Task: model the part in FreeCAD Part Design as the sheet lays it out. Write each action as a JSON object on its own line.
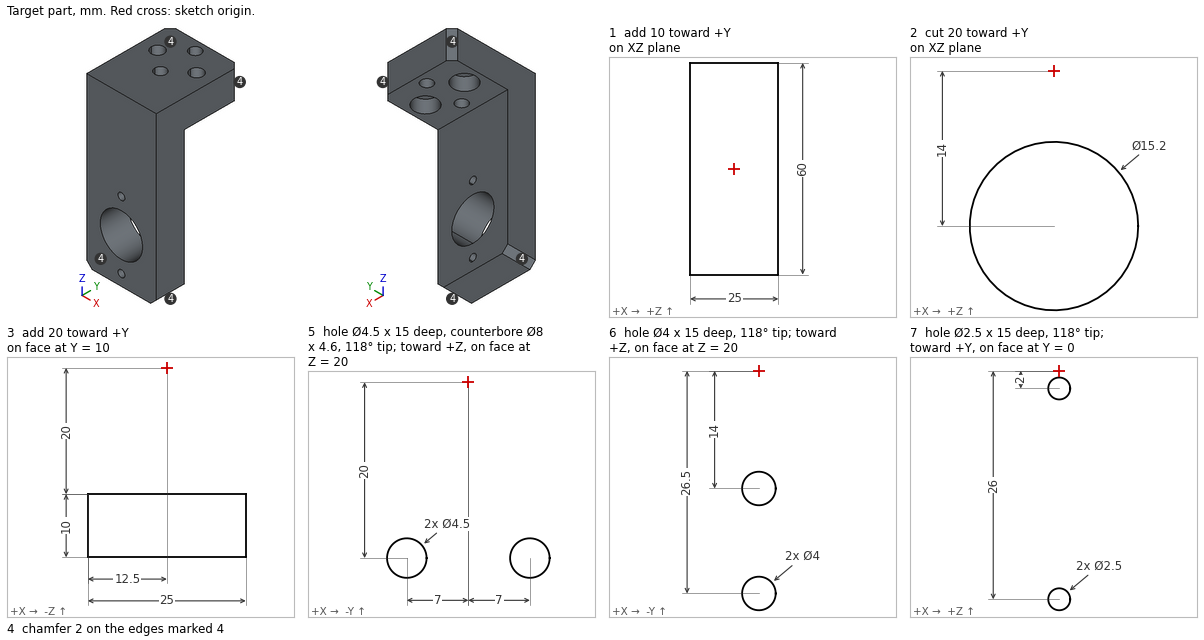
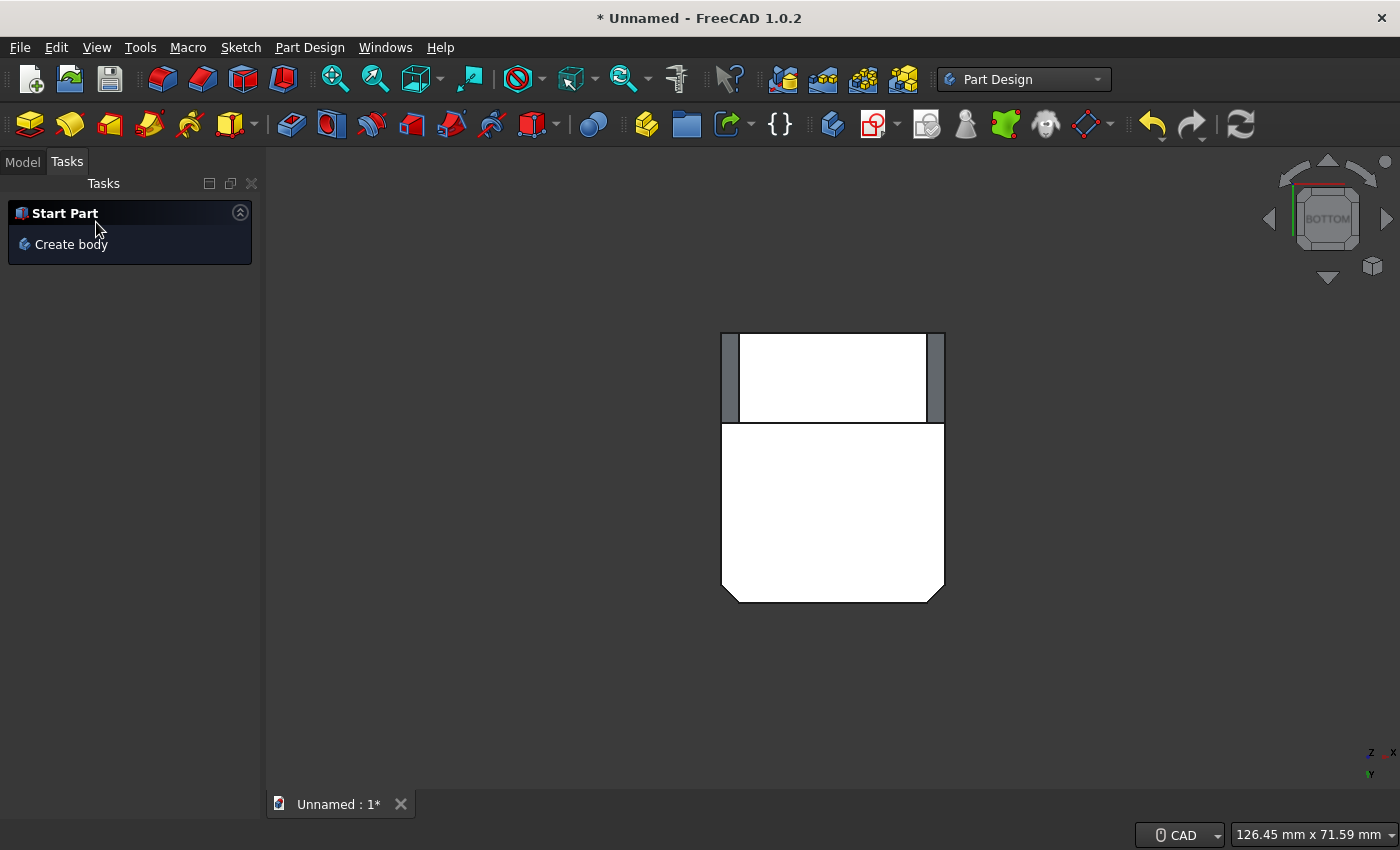
{"action": "left_click", "coordinate": [833, 512]}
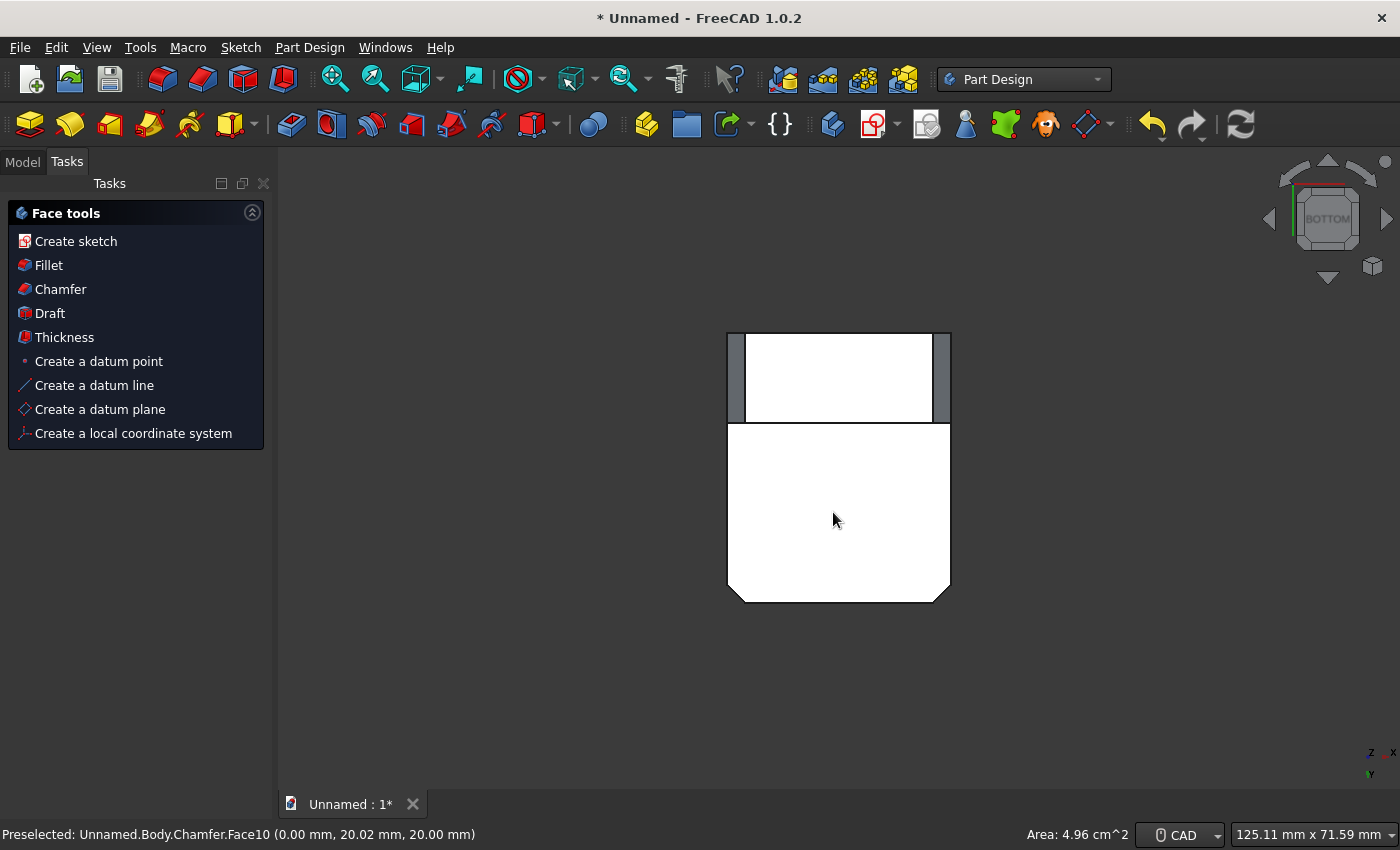
{"action": "left_click", "coordinate": [874, 124]}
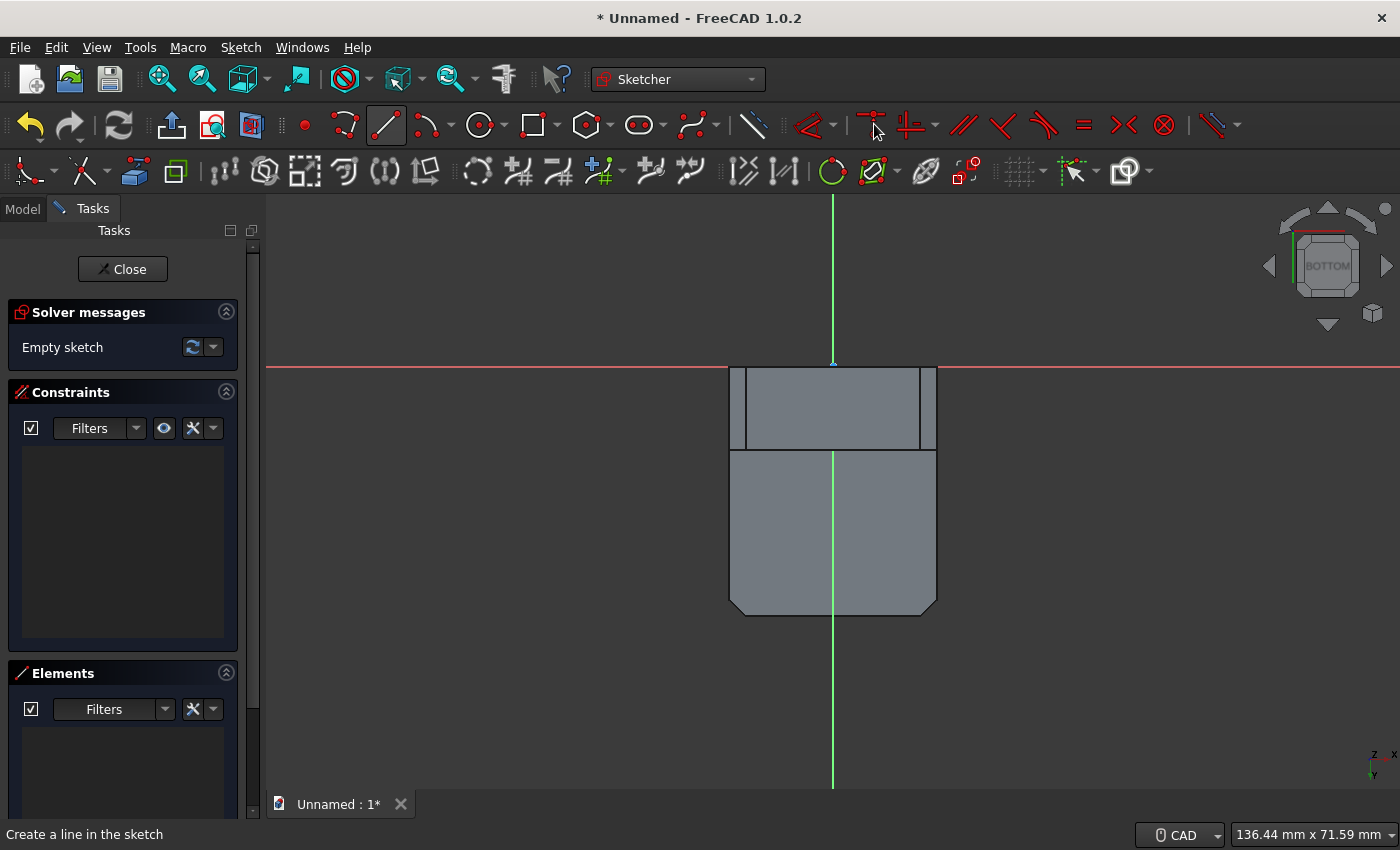
{"action": "key", "text": "q s"}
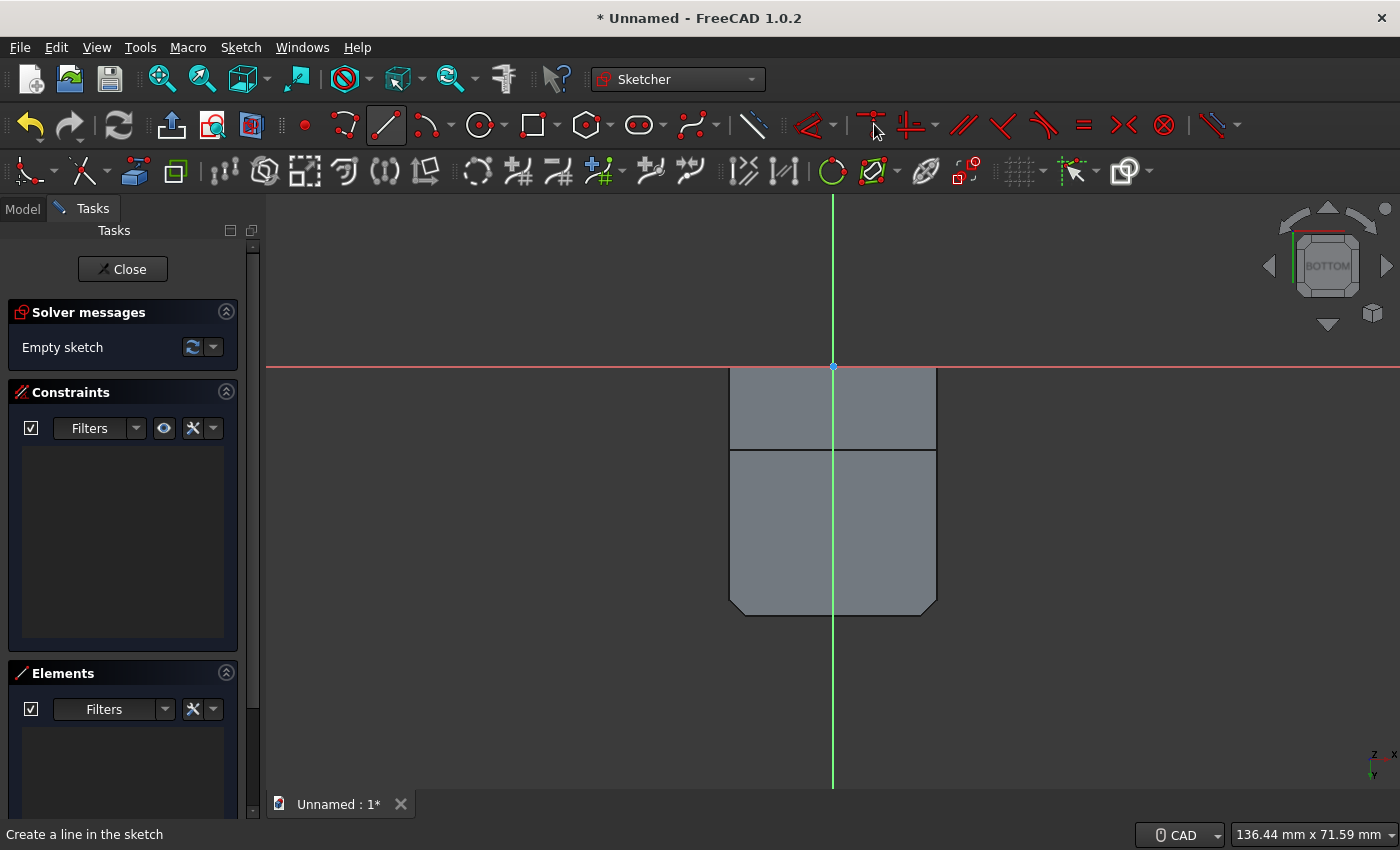
{"action": "scroll", "coordinate": [889, 433], "scroll_direction": "up", "scroll_amount": 4}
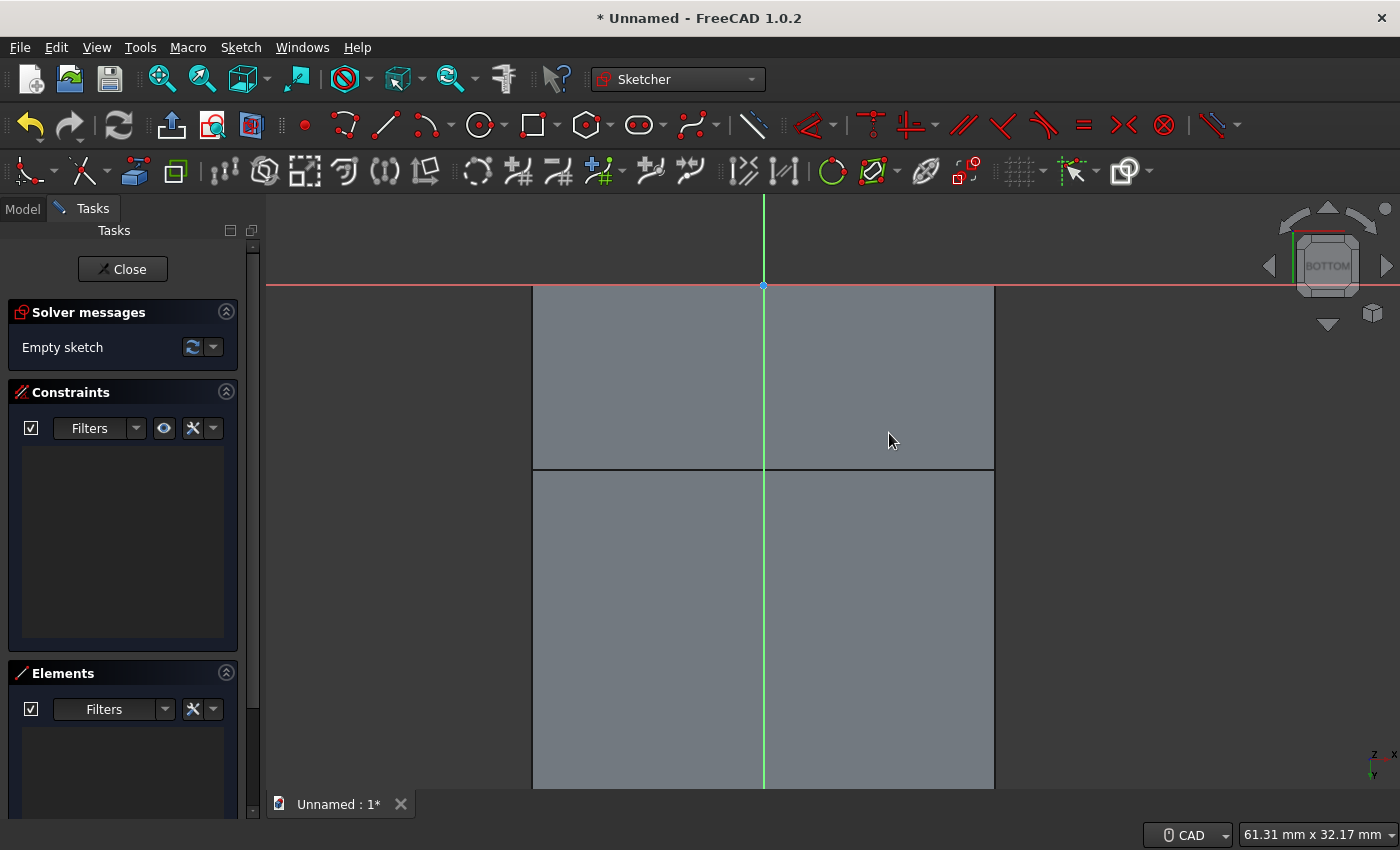
{"action": "key", "text": "g c"}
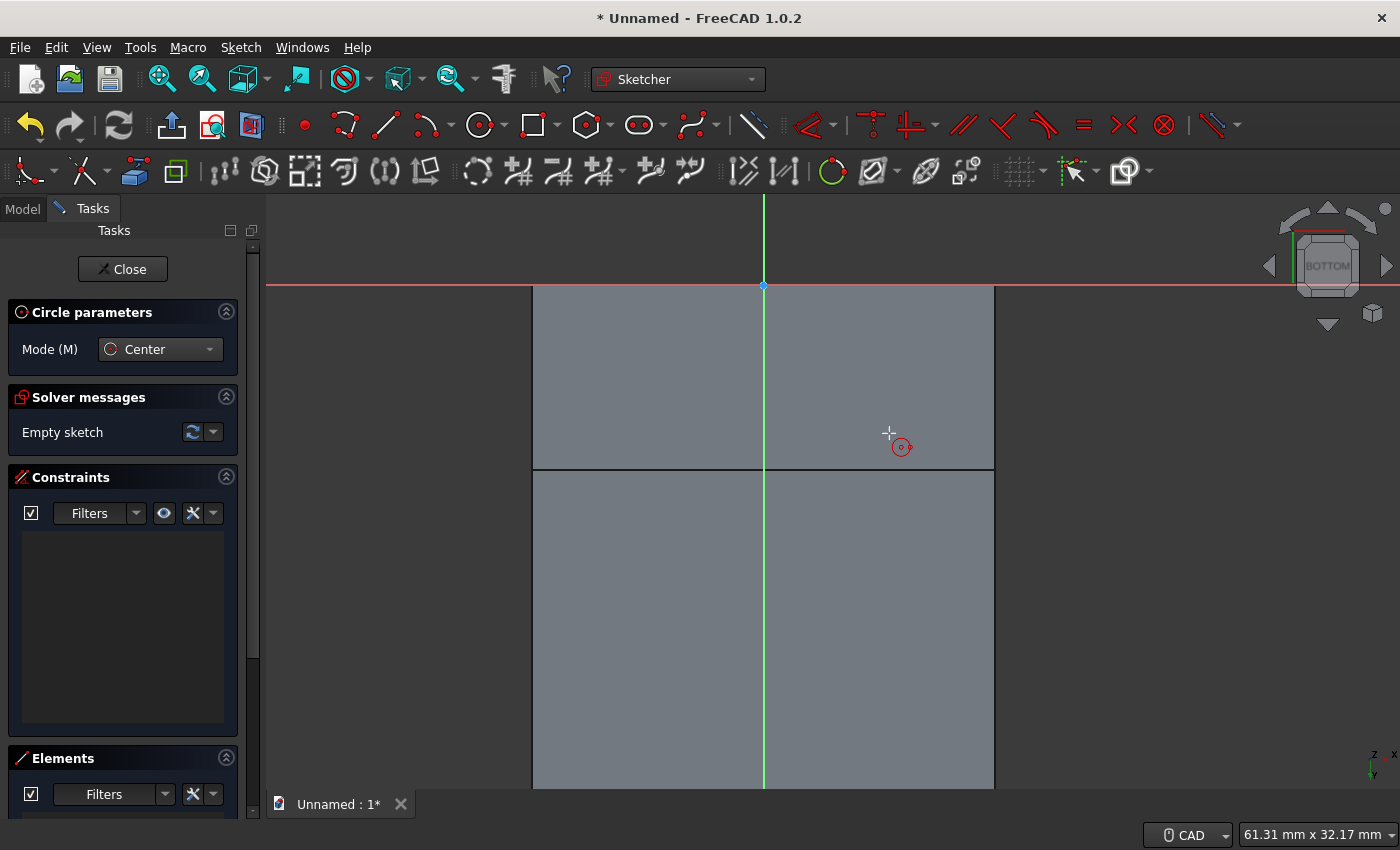
{"action": "left_click", "coordinate": [634, 655]}
{"action": "left_click", "coordinate": [664, 626]}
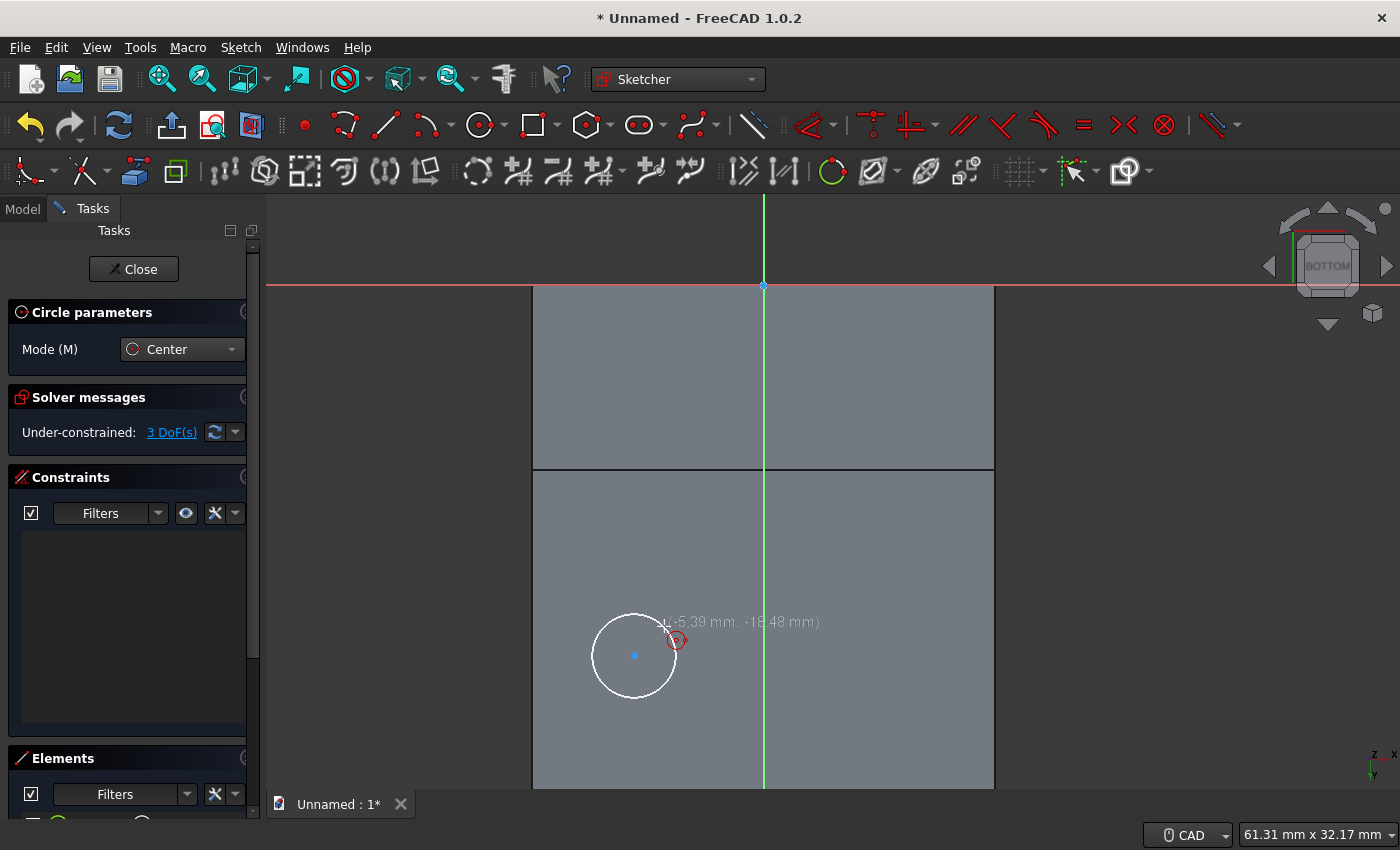
{"action": "left_click", "coordinate": [893, 655]}
{"action": "left_click", "coordinate": [923, 626]}
{"action": "key", "text": "Escape"}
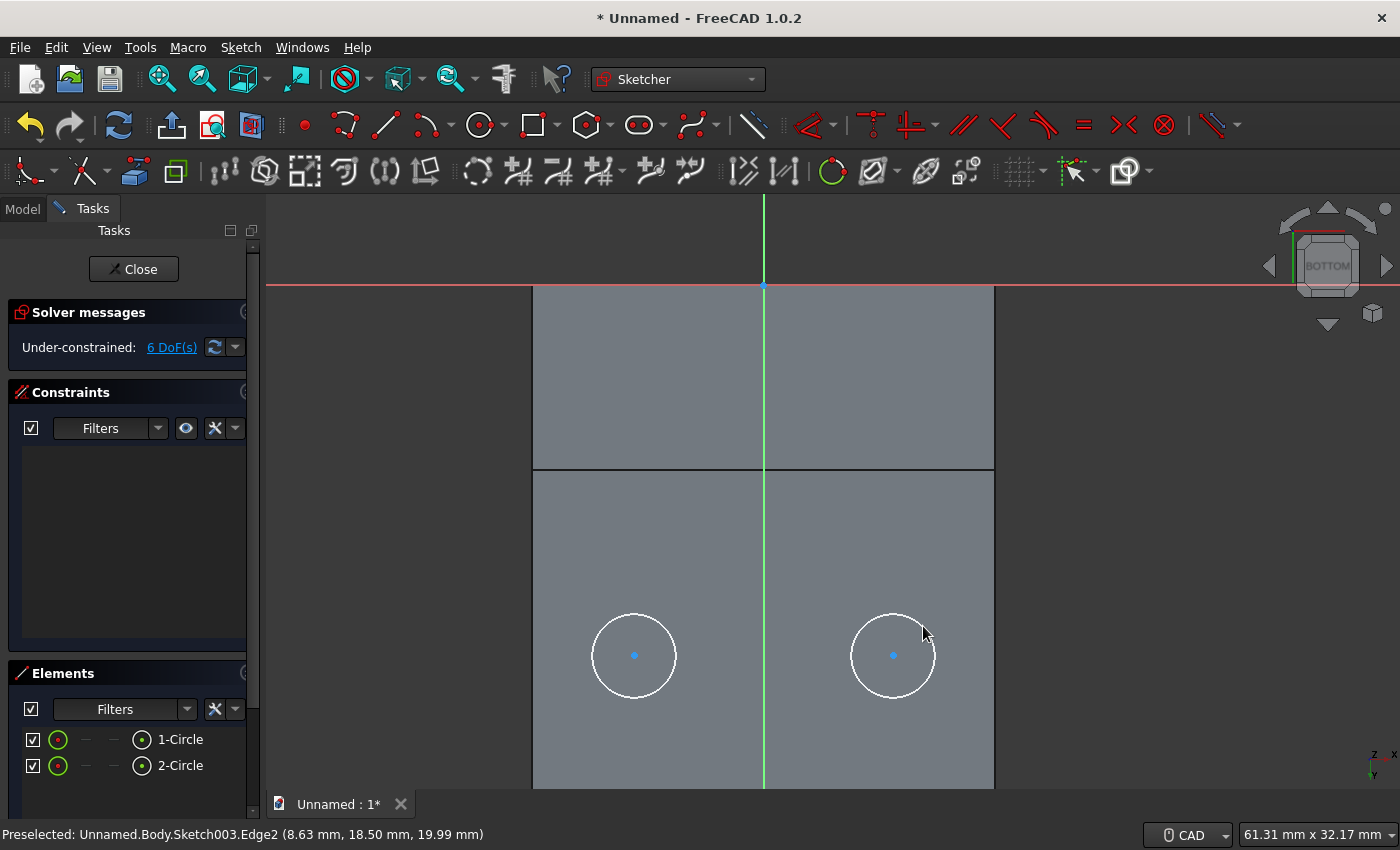
{"action": "left_click", "coordinate": [663, 626]}